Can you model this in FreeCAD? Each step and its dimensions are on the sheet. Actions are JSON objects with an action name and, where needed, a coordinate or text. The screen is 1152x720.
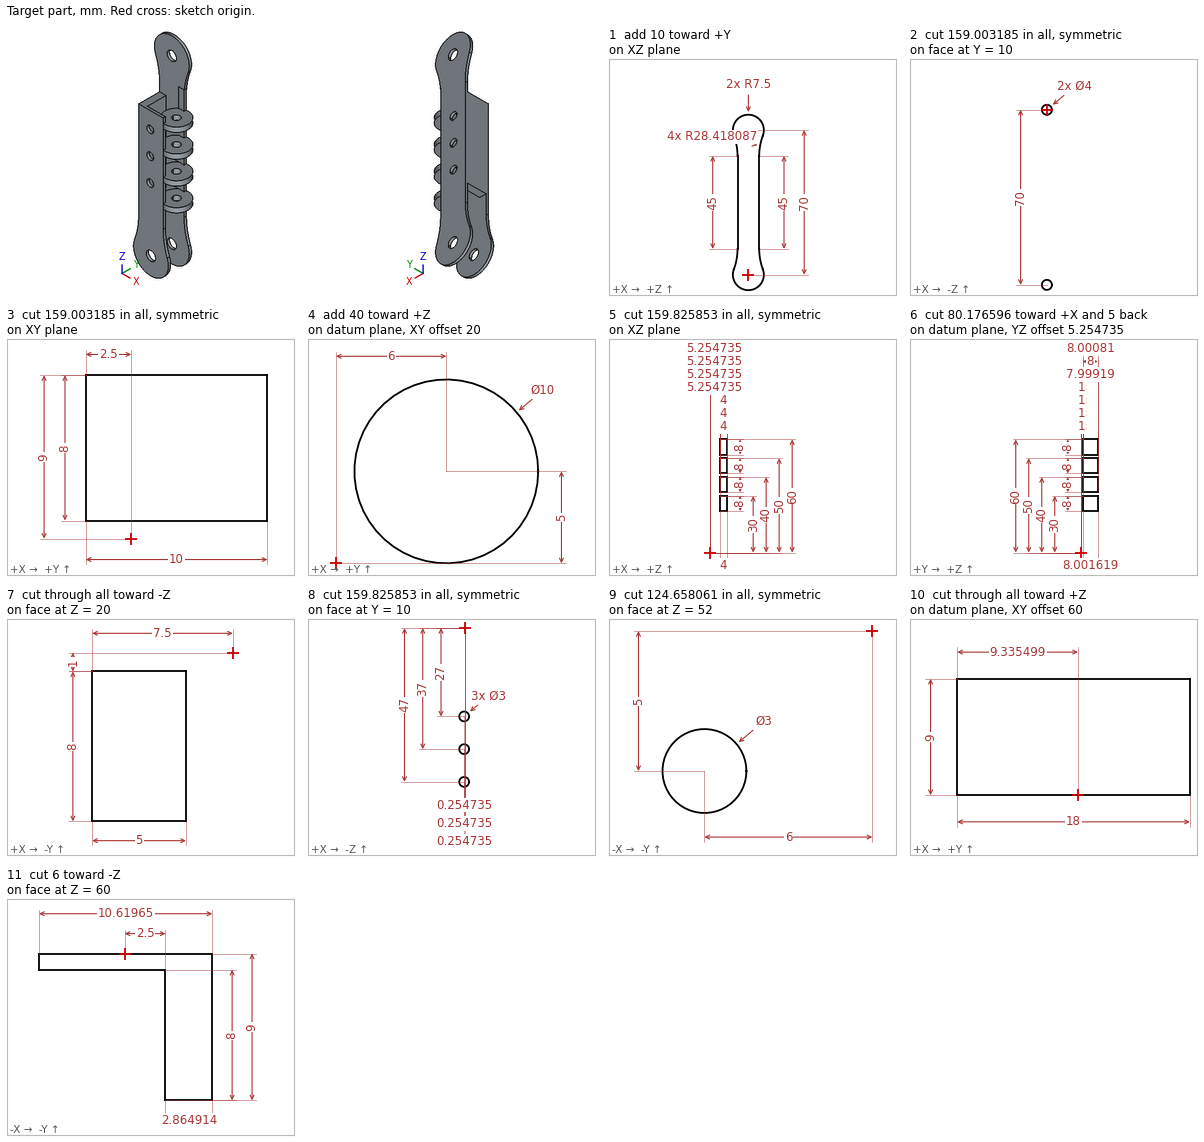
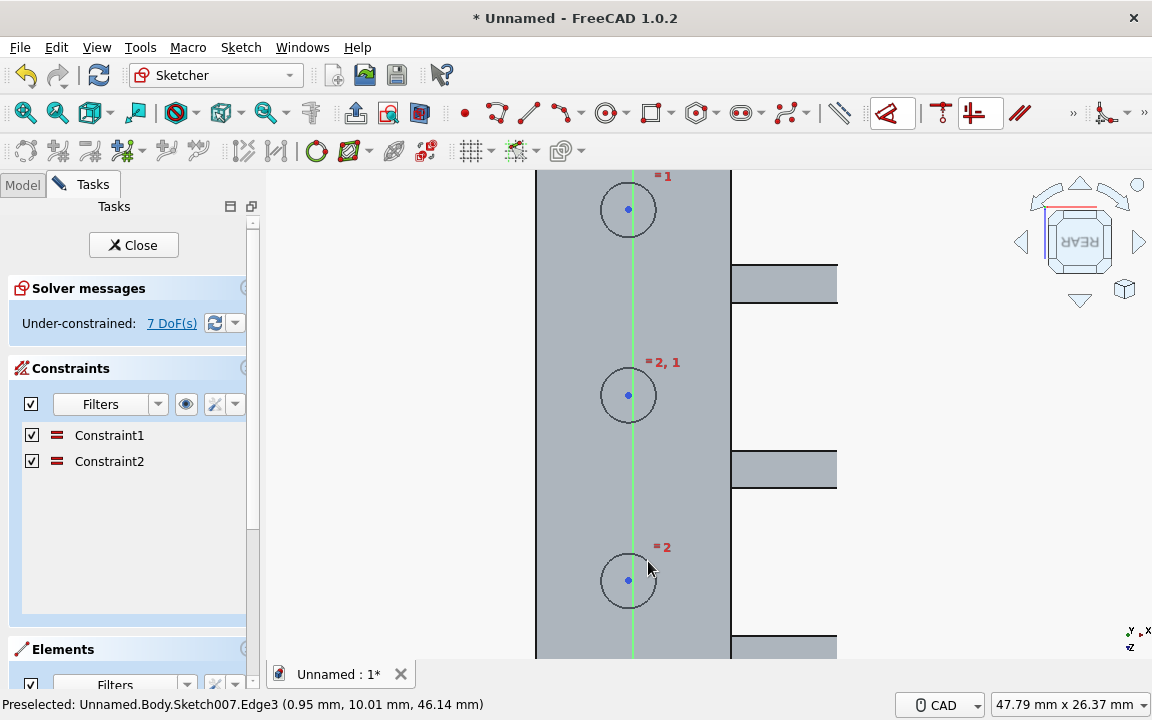
{"action": "left_click", "coordinate": [609, 229]}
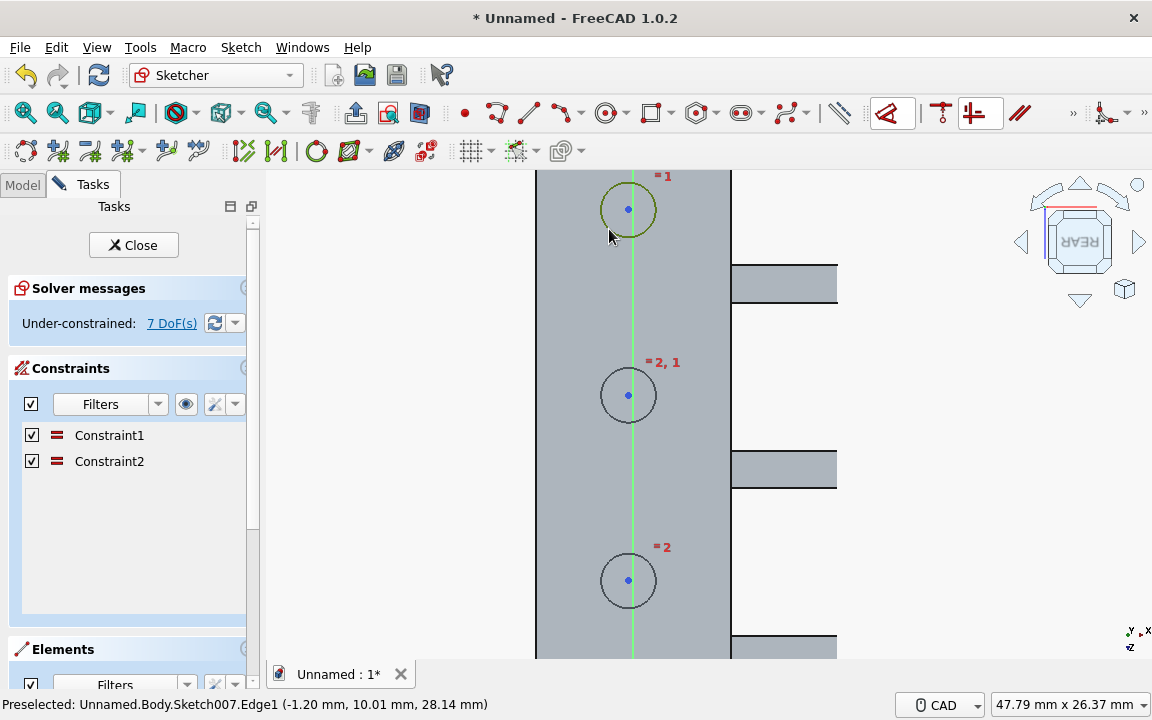
{"action": "left_click", "coordinate": [910, 114]}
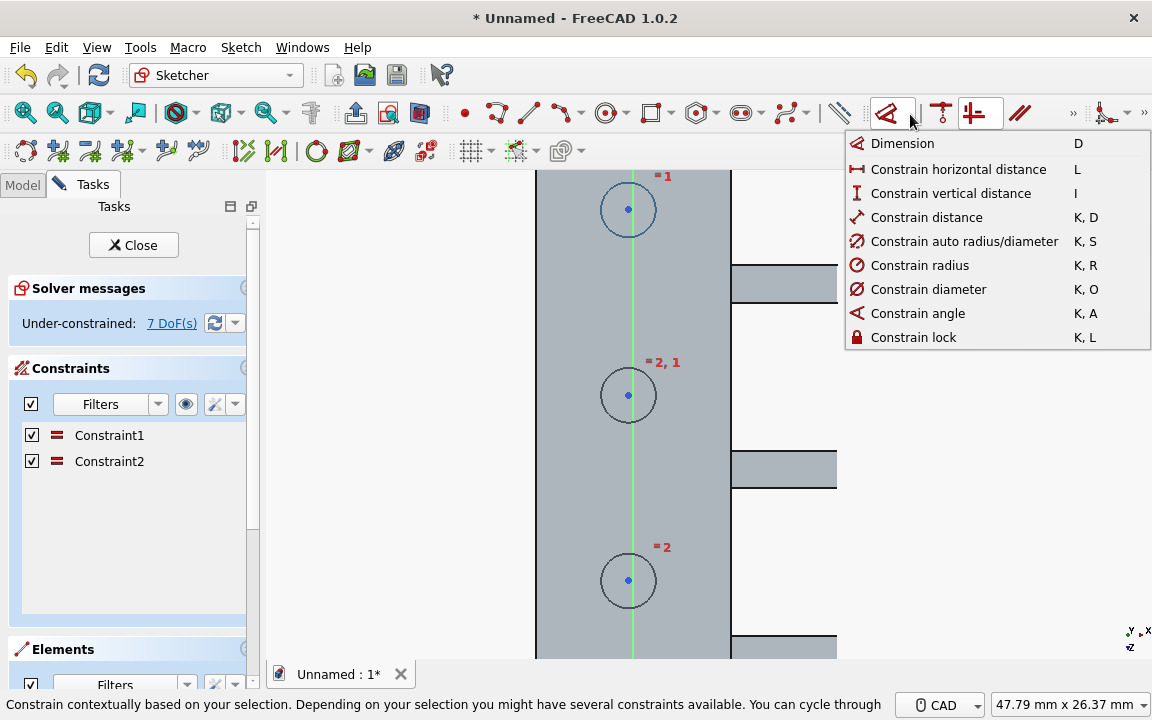
{"action": "left_click", "coordinate": [998, 289]}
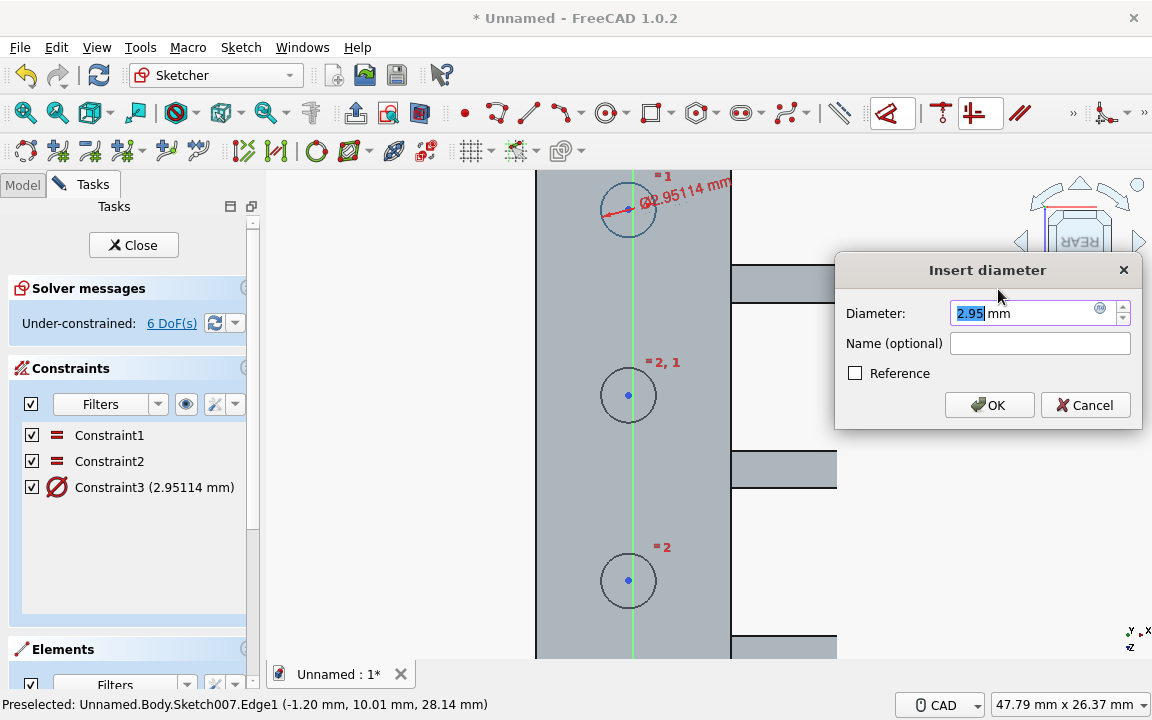
{"action": "type", "text": "3"}
{"action": "key", "text": "Return"}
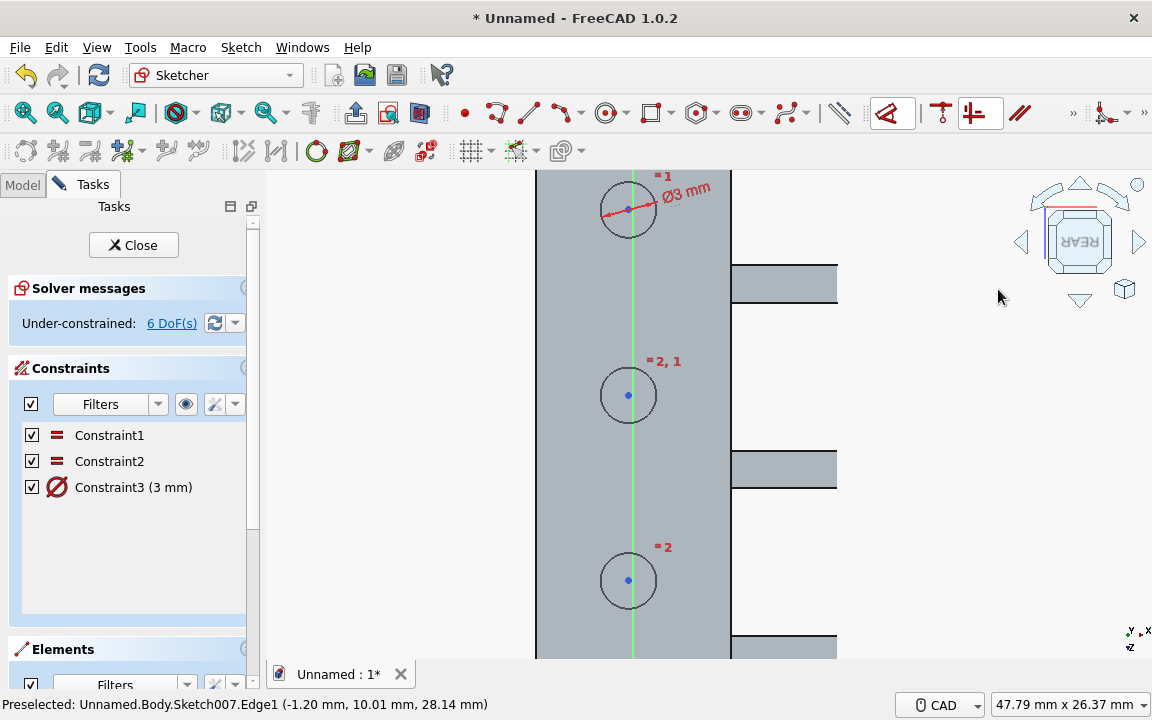
{"action": "left_click", "coordinate": [628, 210]}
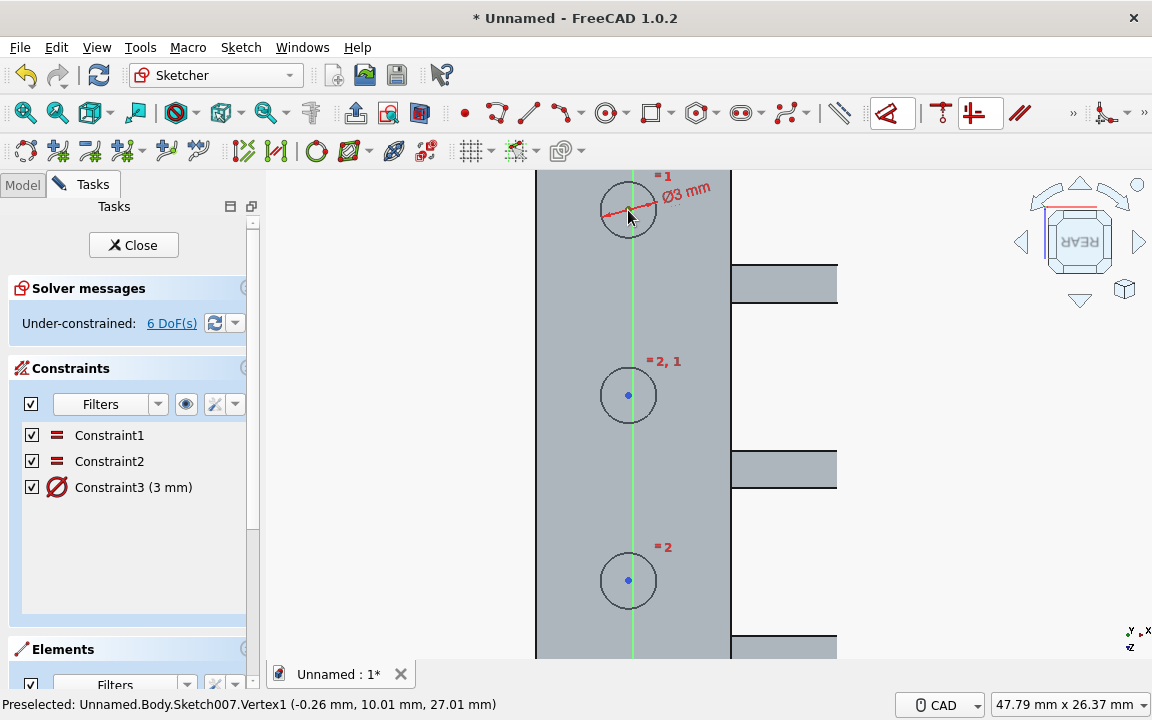
{"action": "left_click", "coordinate": [910, 114]}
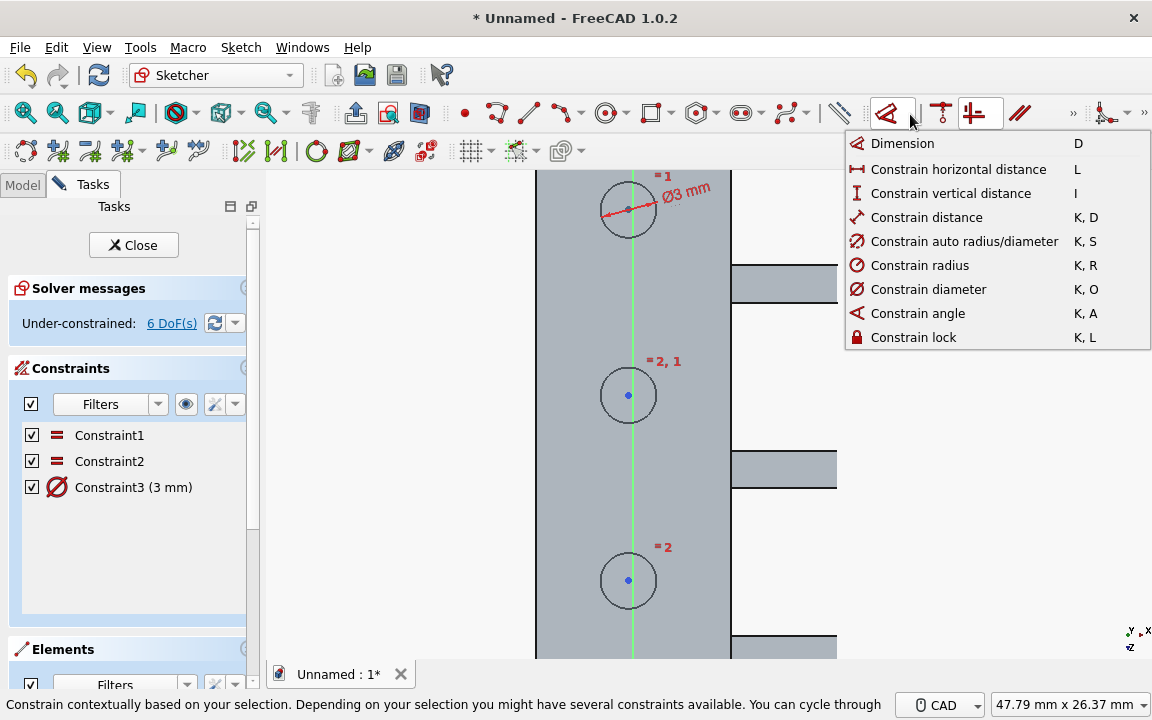
{"action": "left_click", "coordinate": [998, 193]}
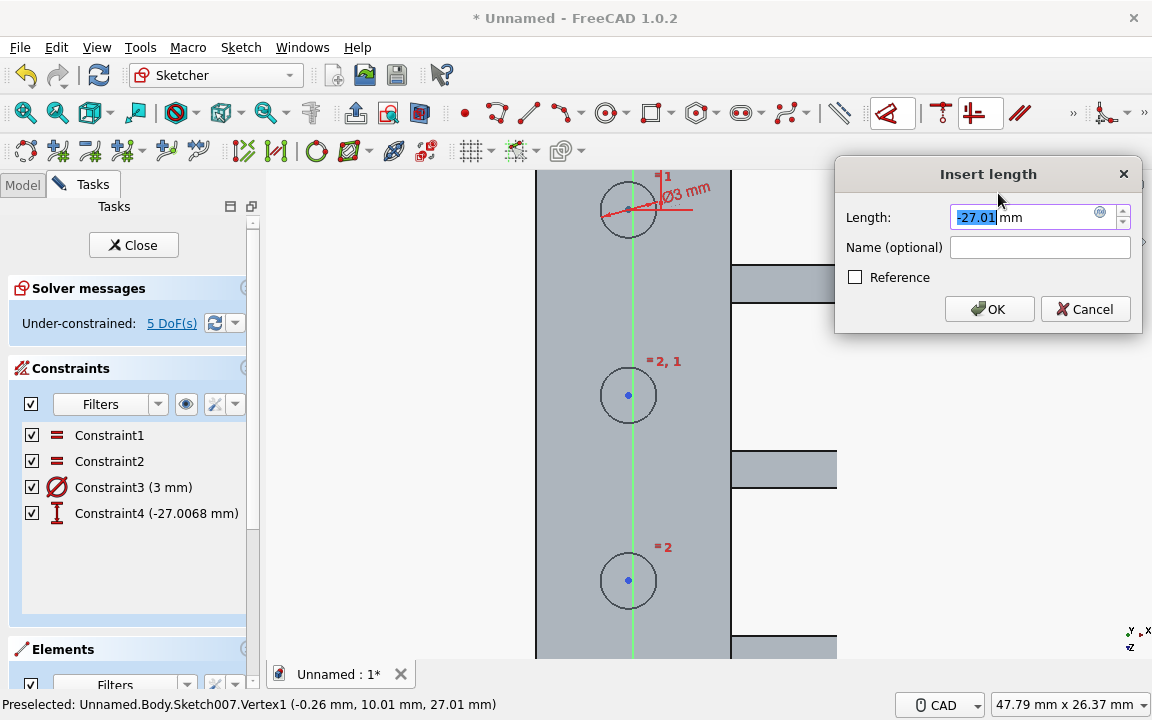
{"action": "type", "text": "-27"}
{"action": "key", "text": "Return"}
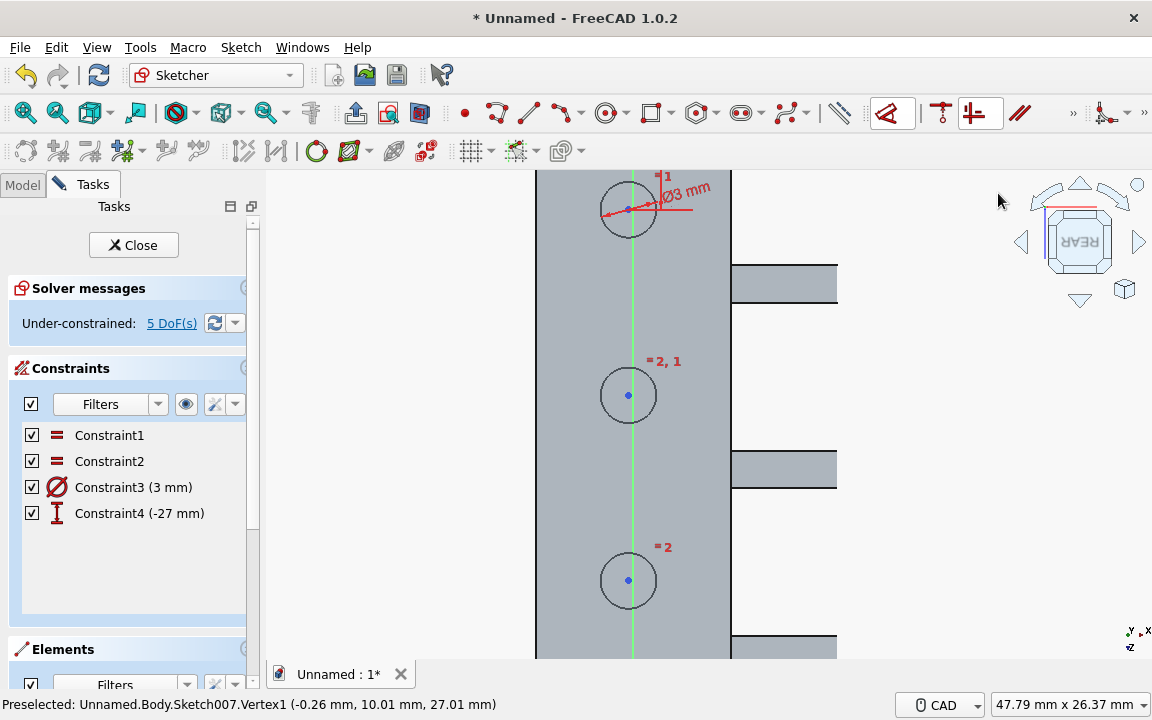
{"action": "left_click", "coordinate": [629, 395]}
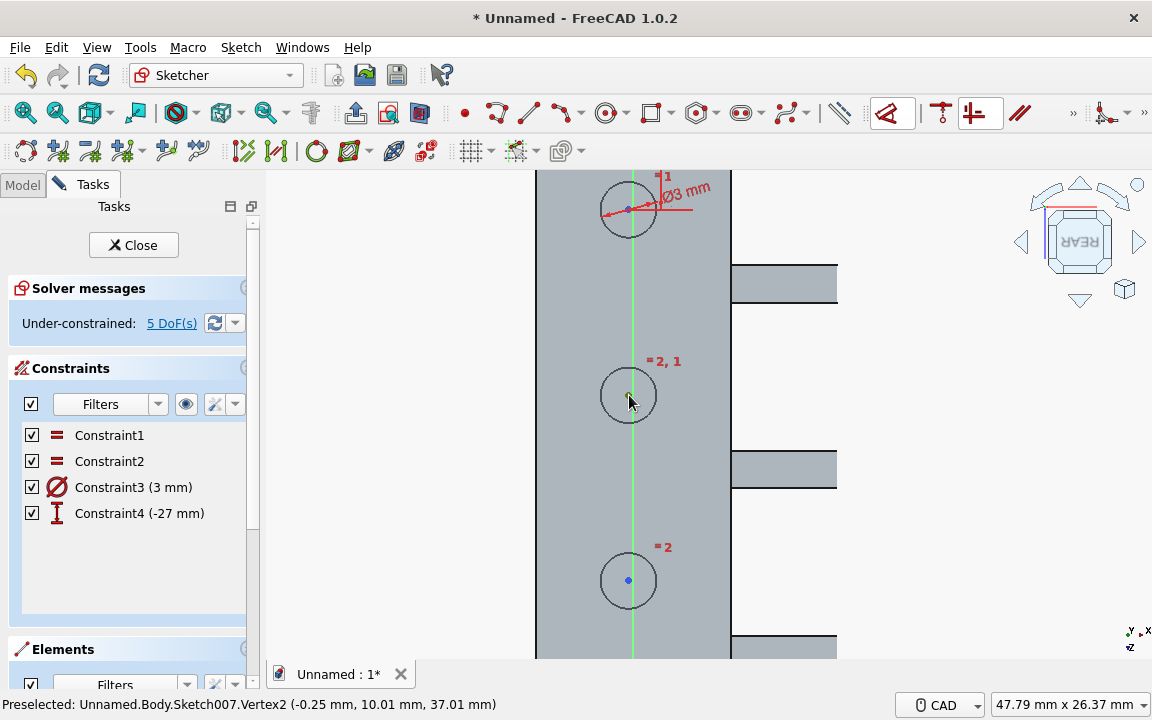
{"action": "left_click", "coordinate": [910, 114]}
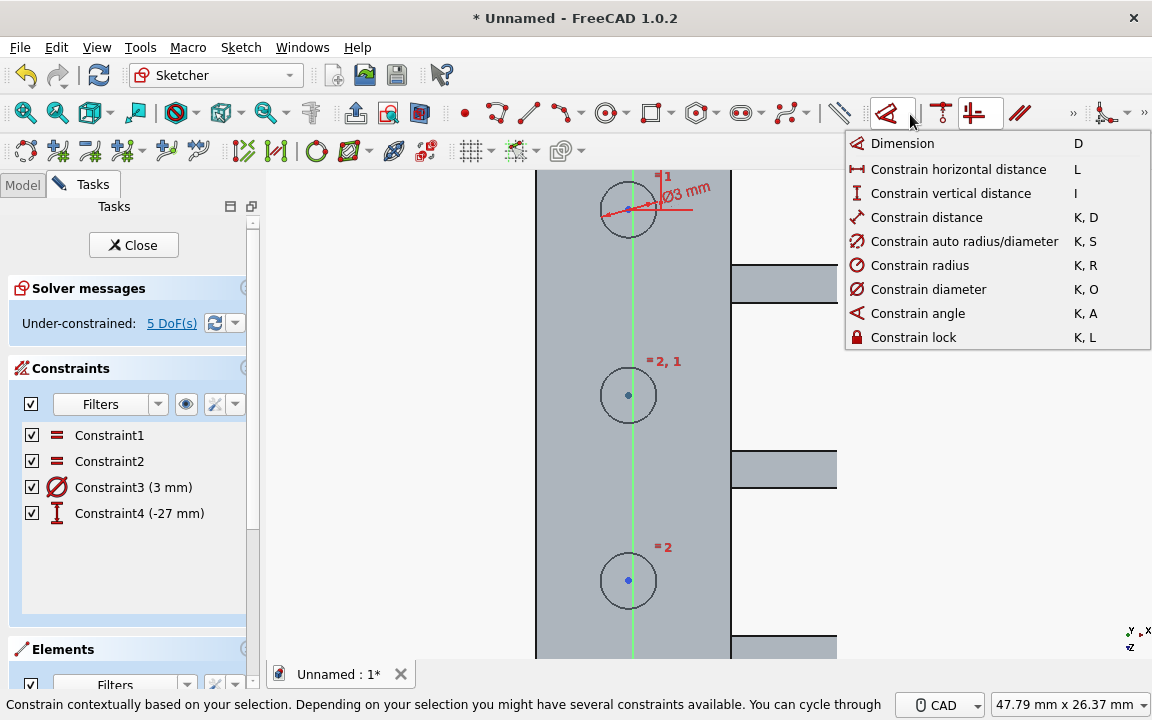
{"action": "left_click", "coordinate": [998, 193]}